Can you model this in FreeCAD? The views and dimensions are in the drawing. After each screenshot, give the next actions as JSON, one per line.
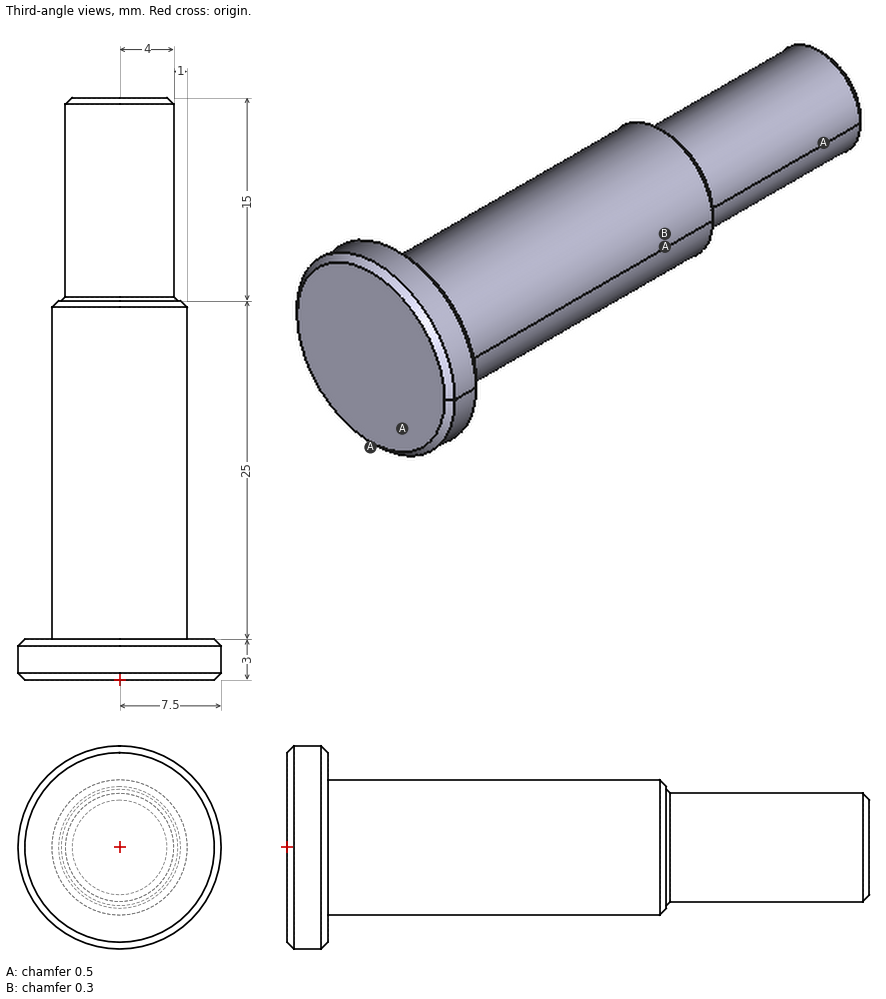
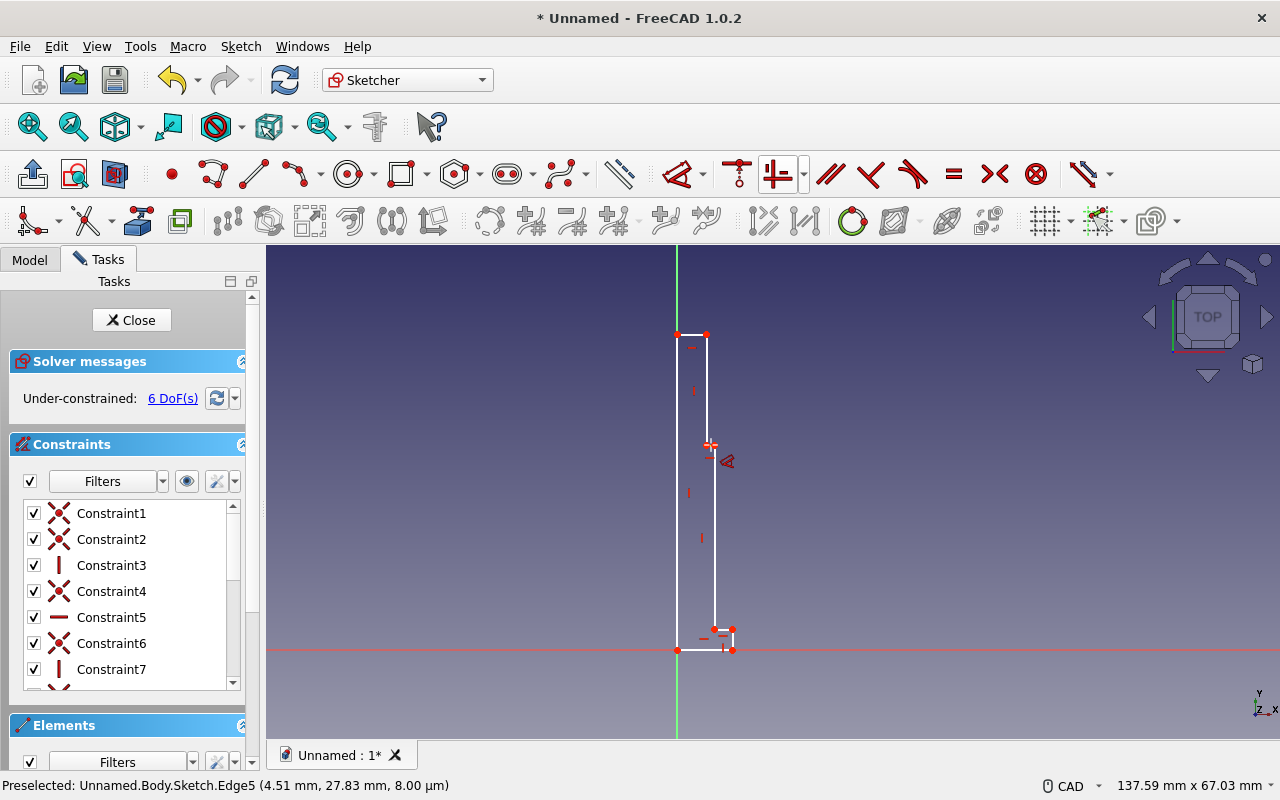
{"action": "scroll", "coordinate": [733, 644], "scroll_direction": "up", "scroll_amount": 4}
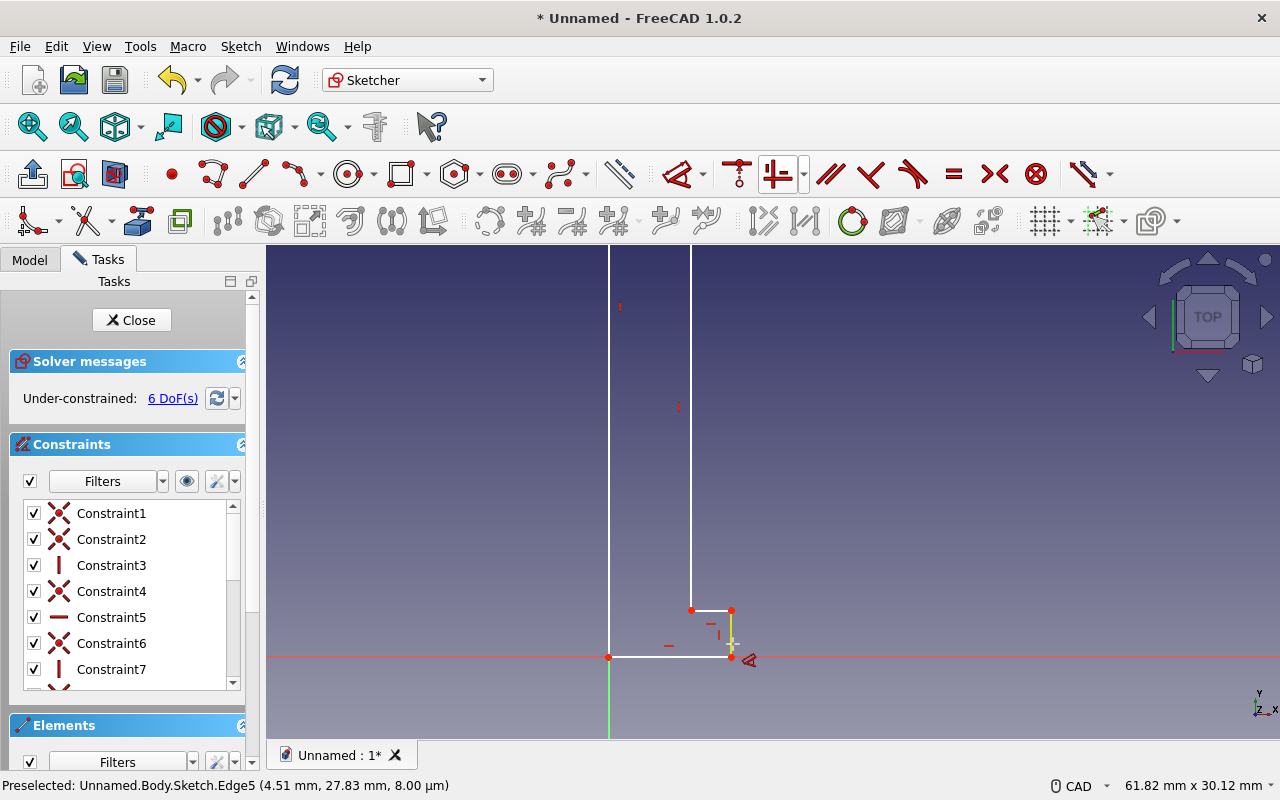
{"action": "left_click", "coordinate": [731, 643]}
{"action": "left_click", "coordinate": [765, 634]}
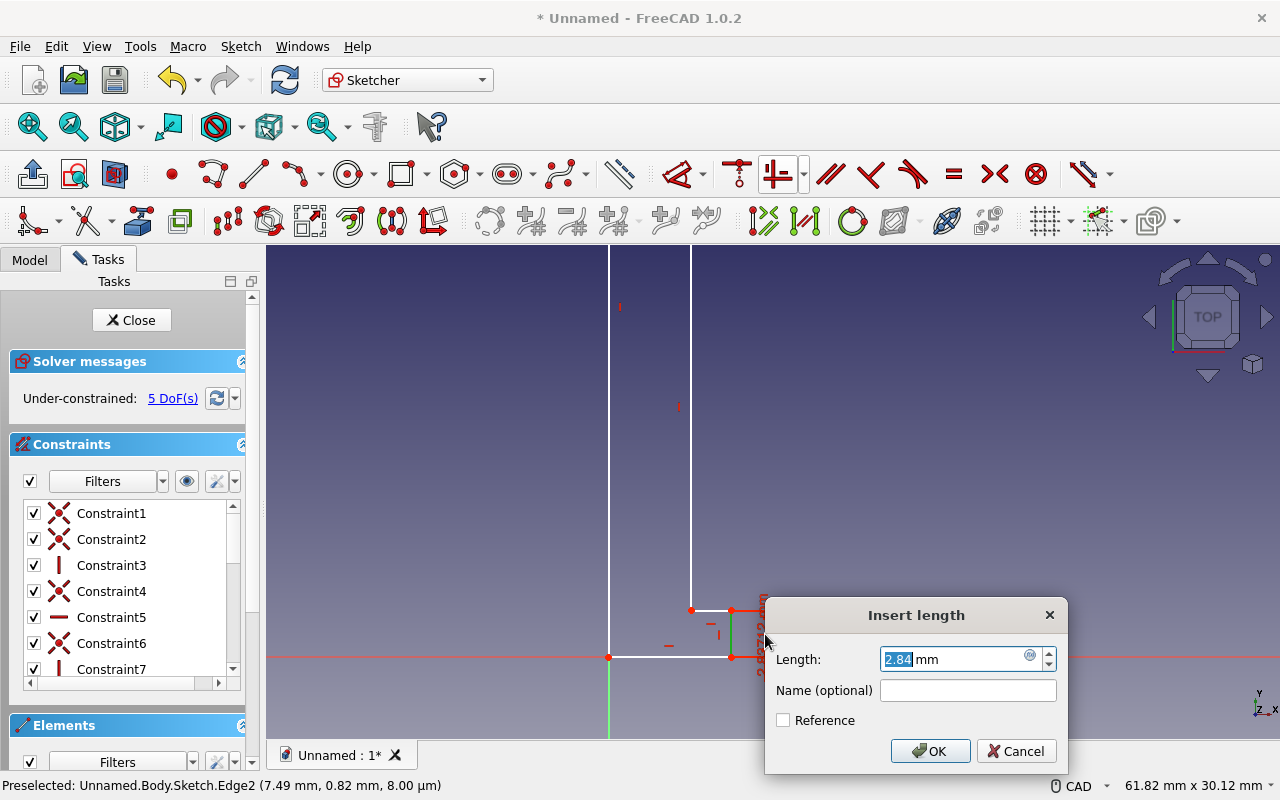
{"action": "type", "text": "3"}
{"action": "key", "text": "Return"}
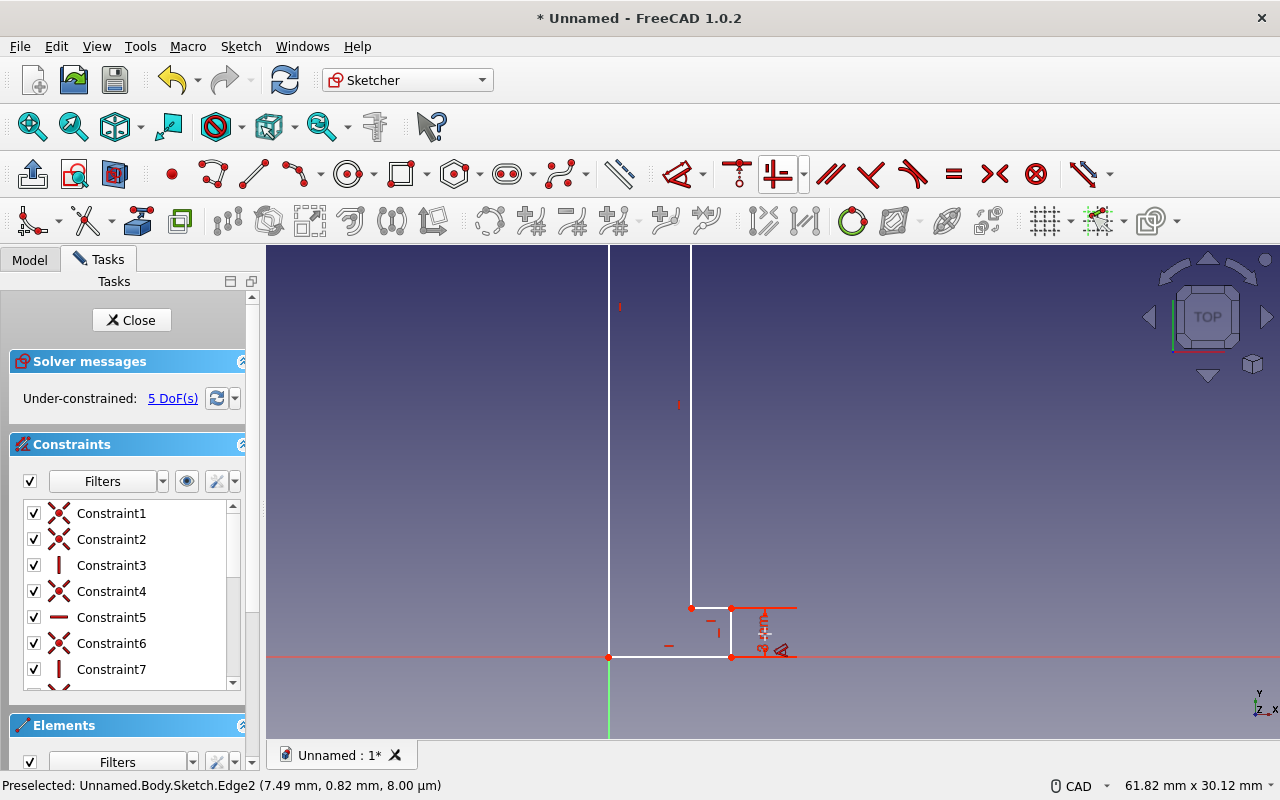
{"action": "scroll", "coordinate": [733, 645], "scroll_direction": "down", "scroll_amount": 4}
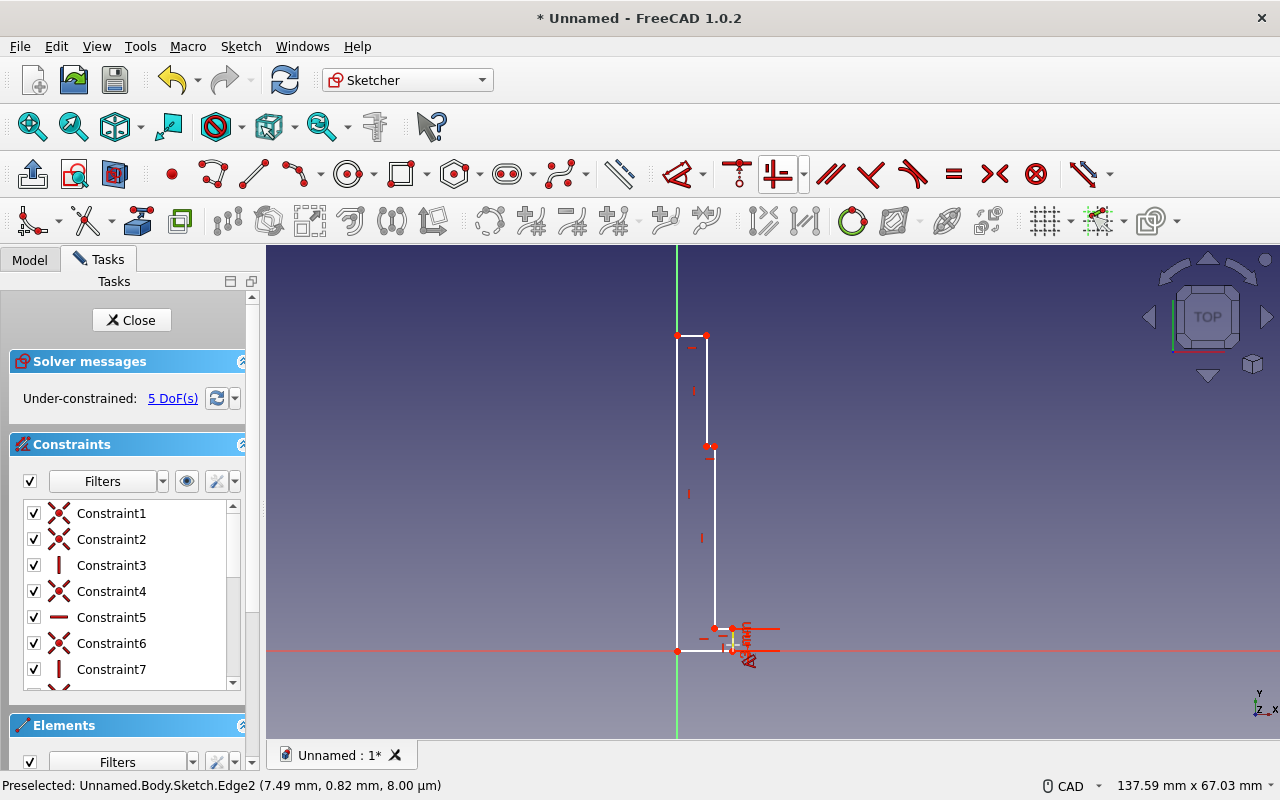
{"action": "scroll", "coordinate": [711, 446], "scroll_direction": "up", "scroll_amount": 9}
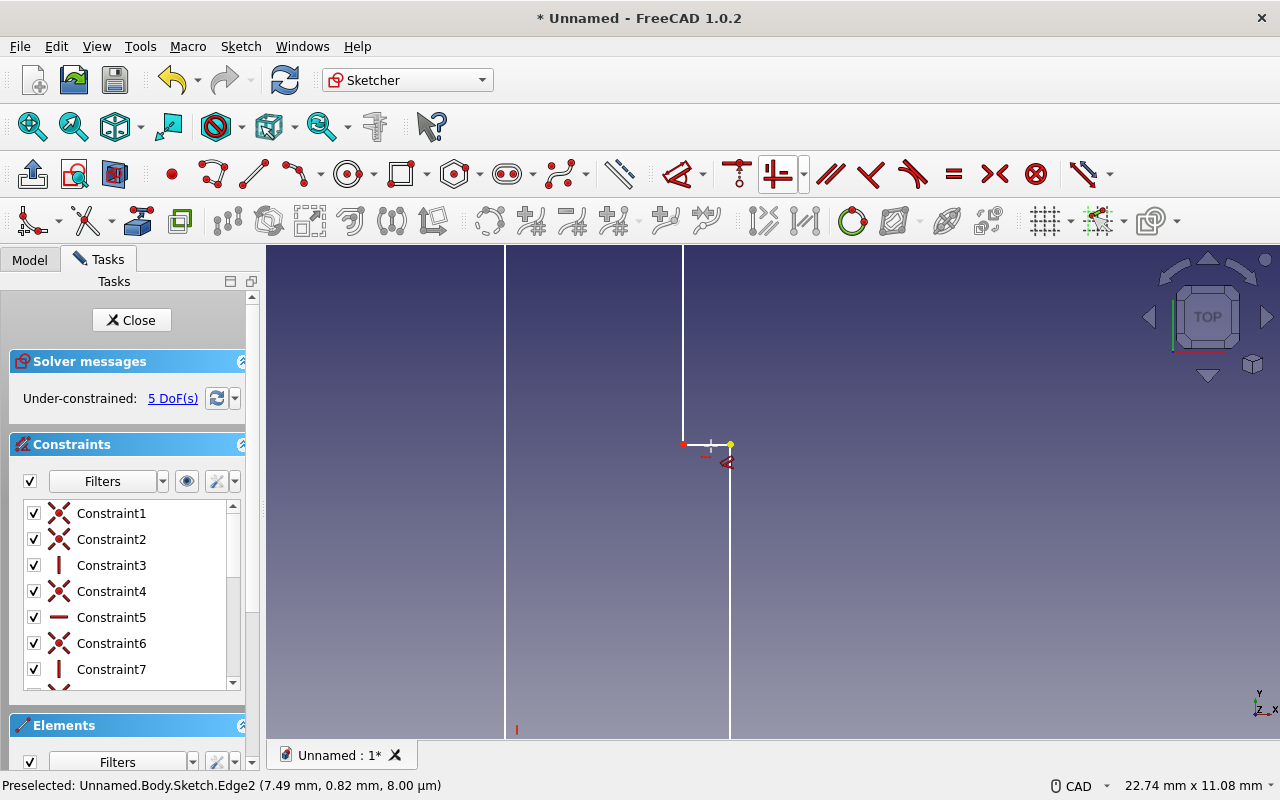
{"action": "left_click", "coordinate": [707, 445]}
{"action": "left_click", "coordinate": [707, 411]}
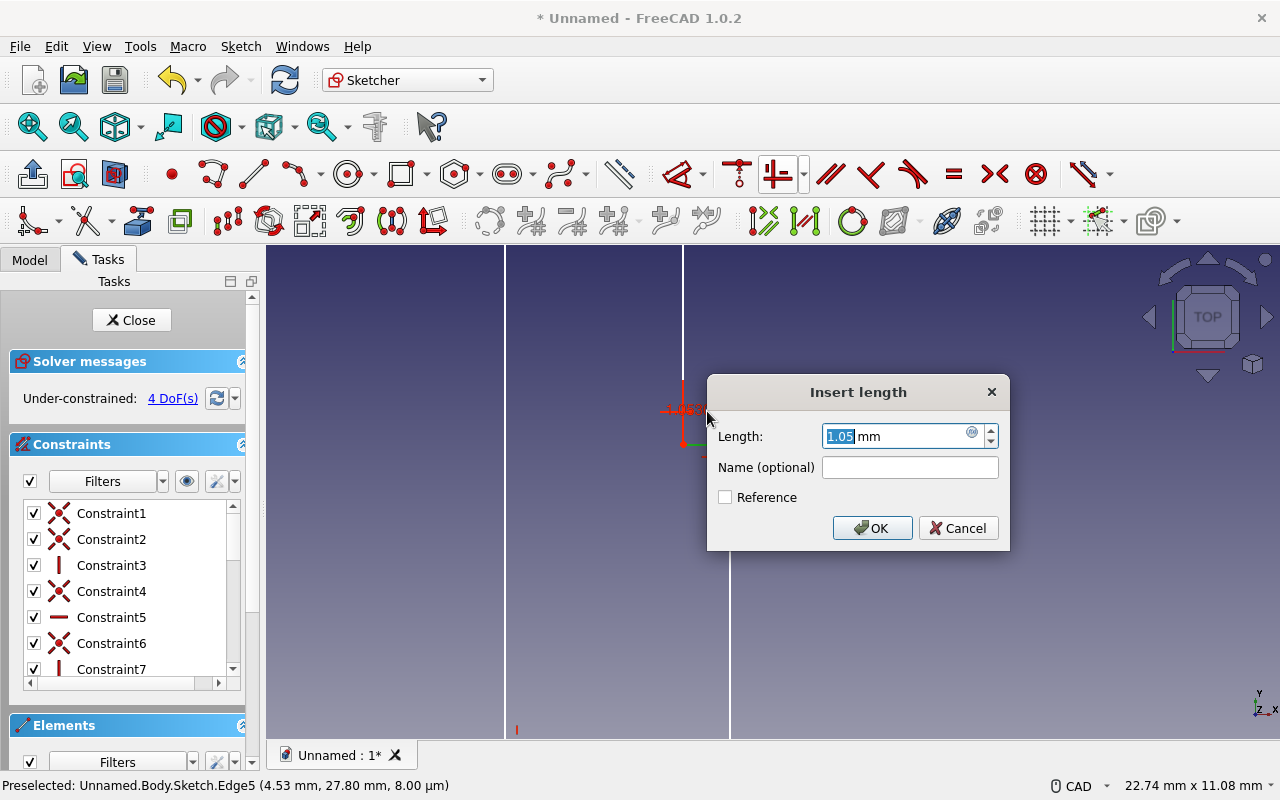
{"action": "type", "text": "1"}
{"action": "key", "text": "Return"}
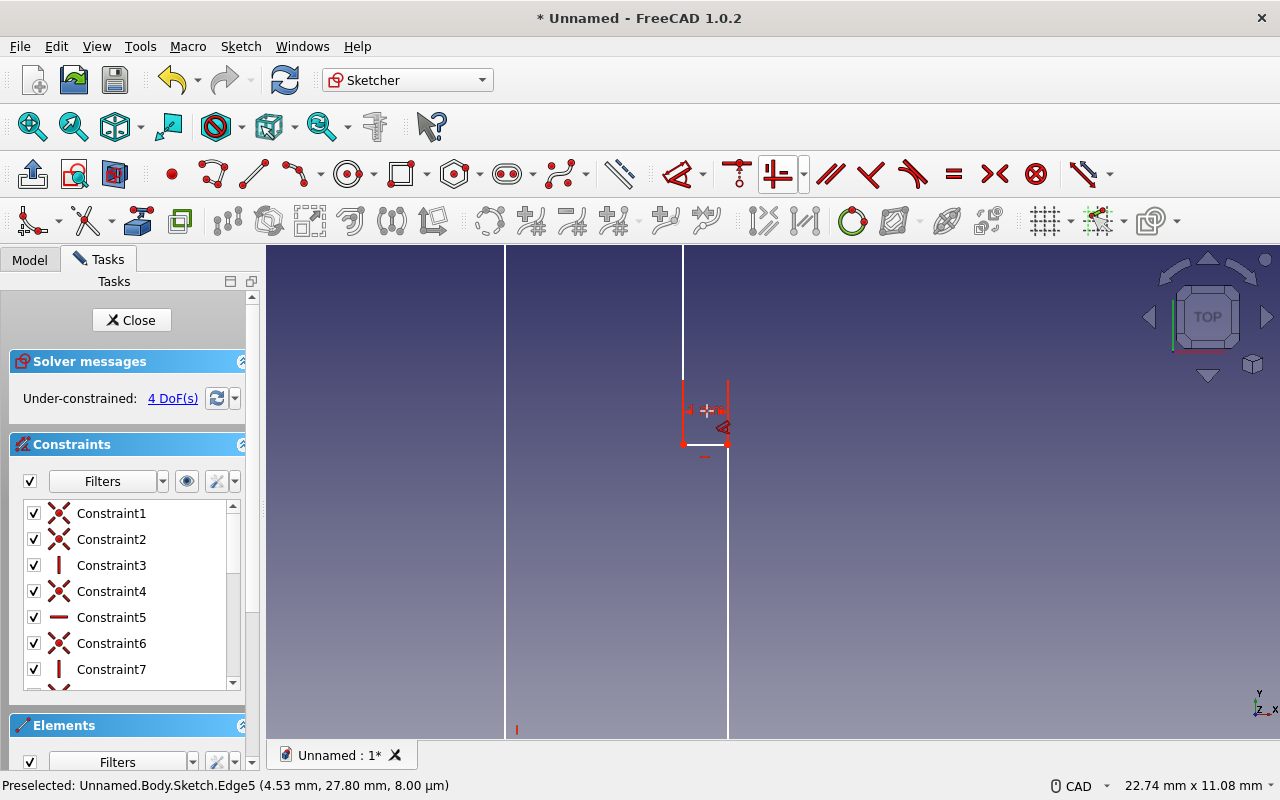
{"action": "scroll", "coordinate": [711, 446], "scroll_direction": "down", "scroll_amount": 9}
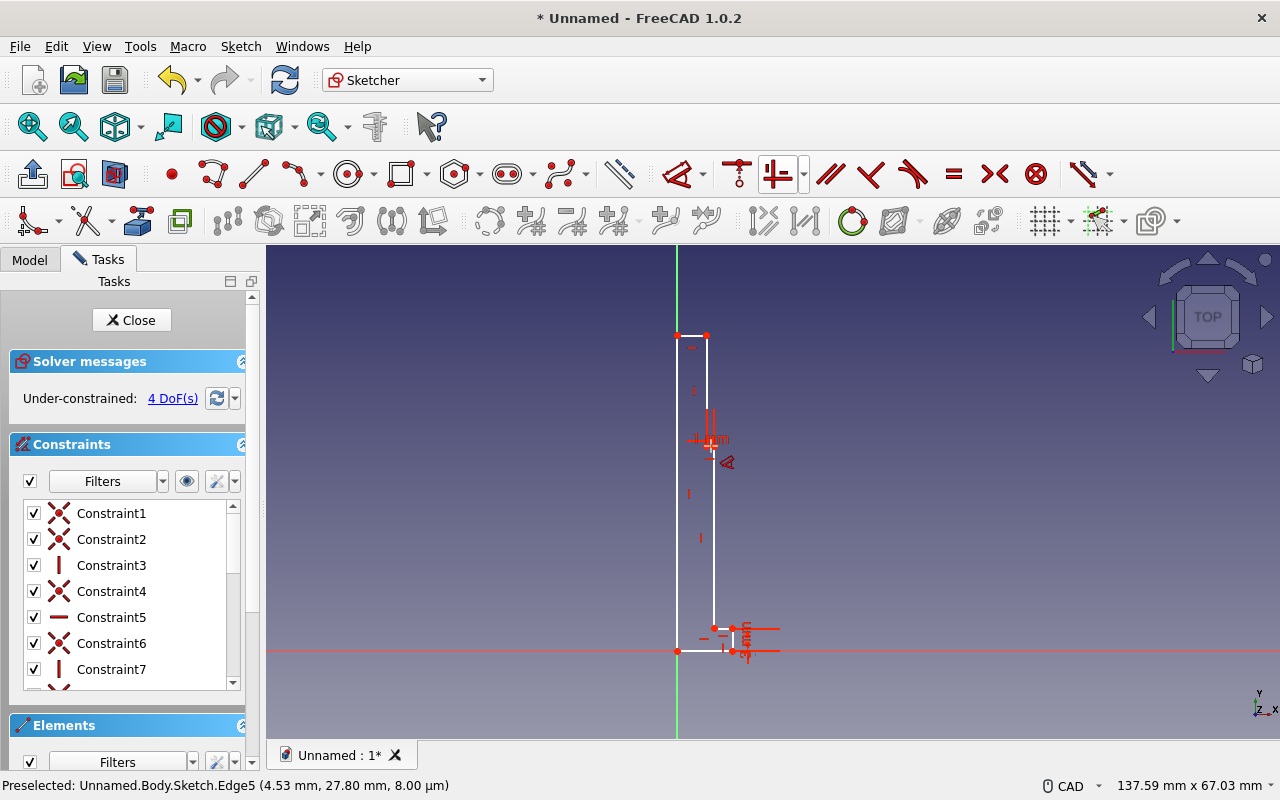
{"action": "scroll", "coordinate": [698, 336], "scroll_direction": "up", "scroll_amount": 3}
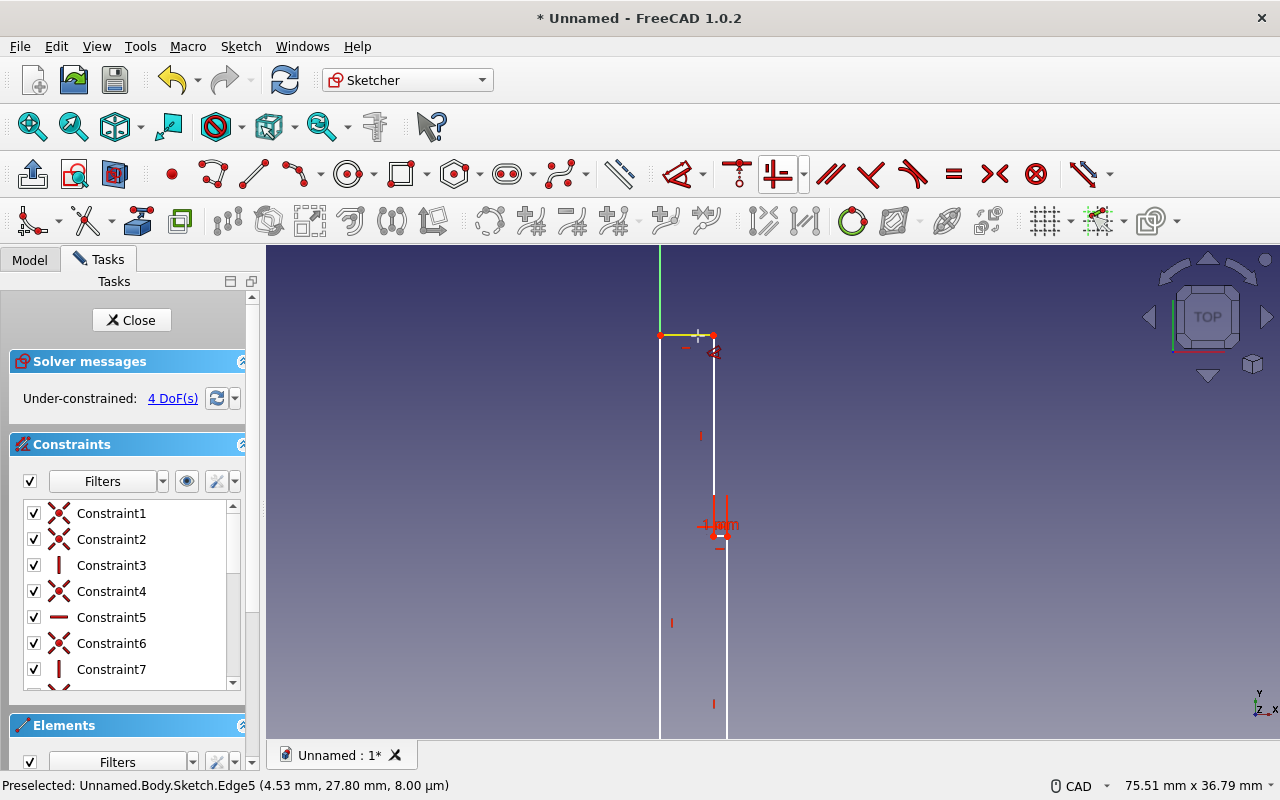
{"action": "left_click", "coordinate": [698, 335]}
{"action": "left_click", "coordinate": [687, 301]}